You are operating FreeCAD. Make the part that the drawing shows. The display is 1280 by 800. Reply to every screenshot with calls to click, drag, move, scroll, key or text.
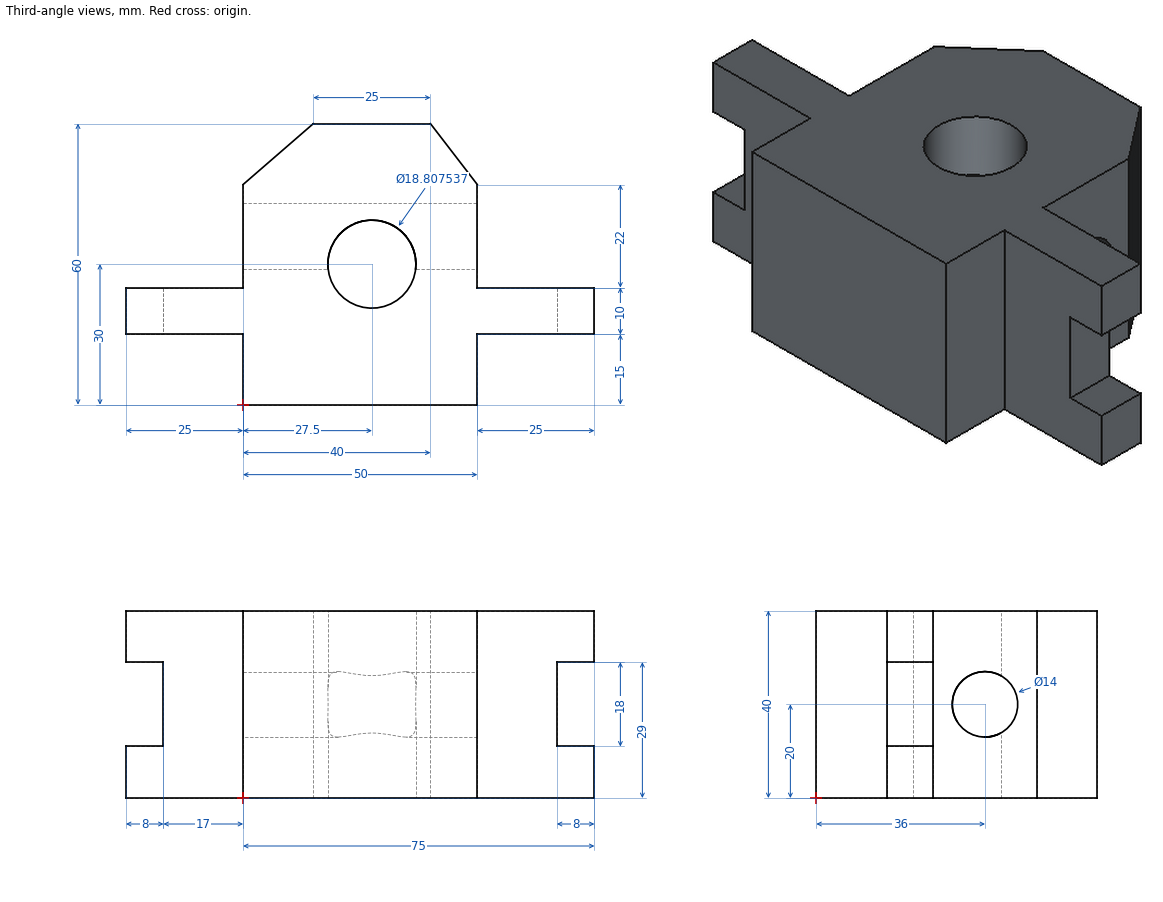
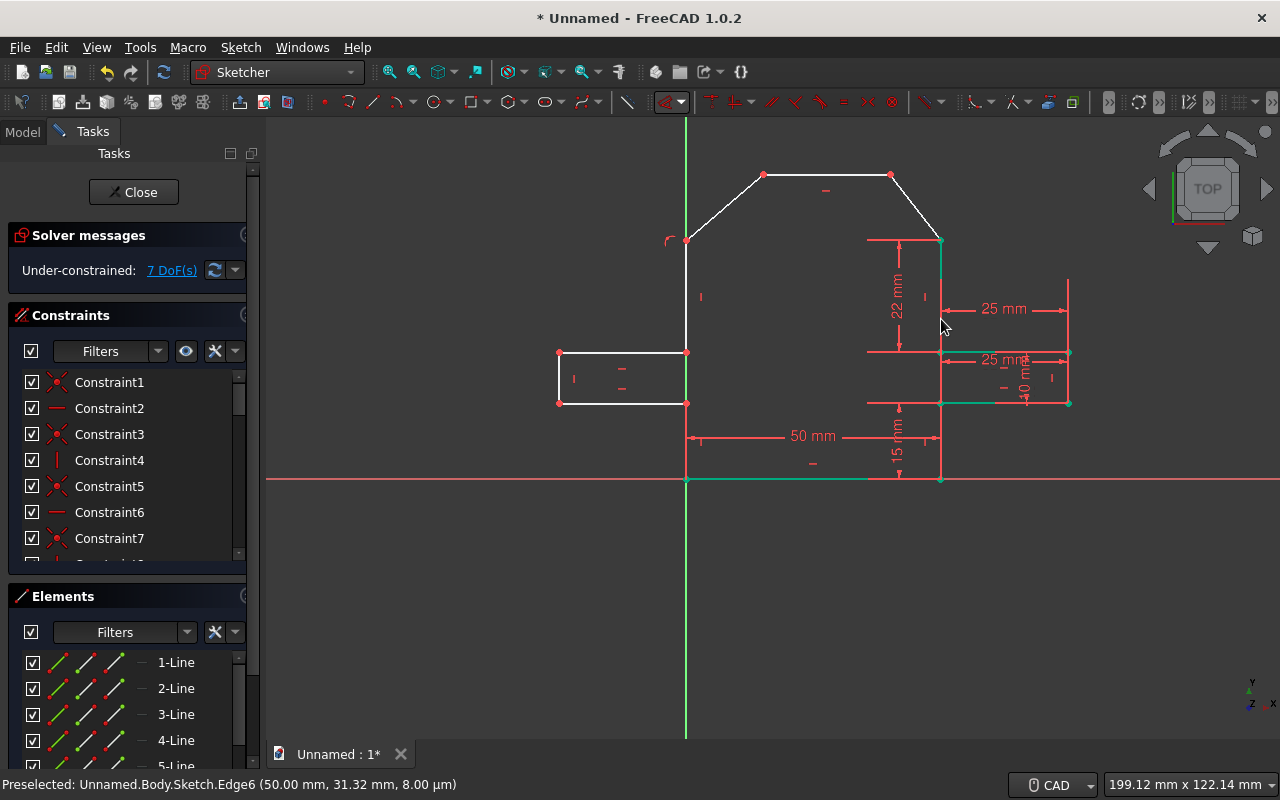
click(852, 175)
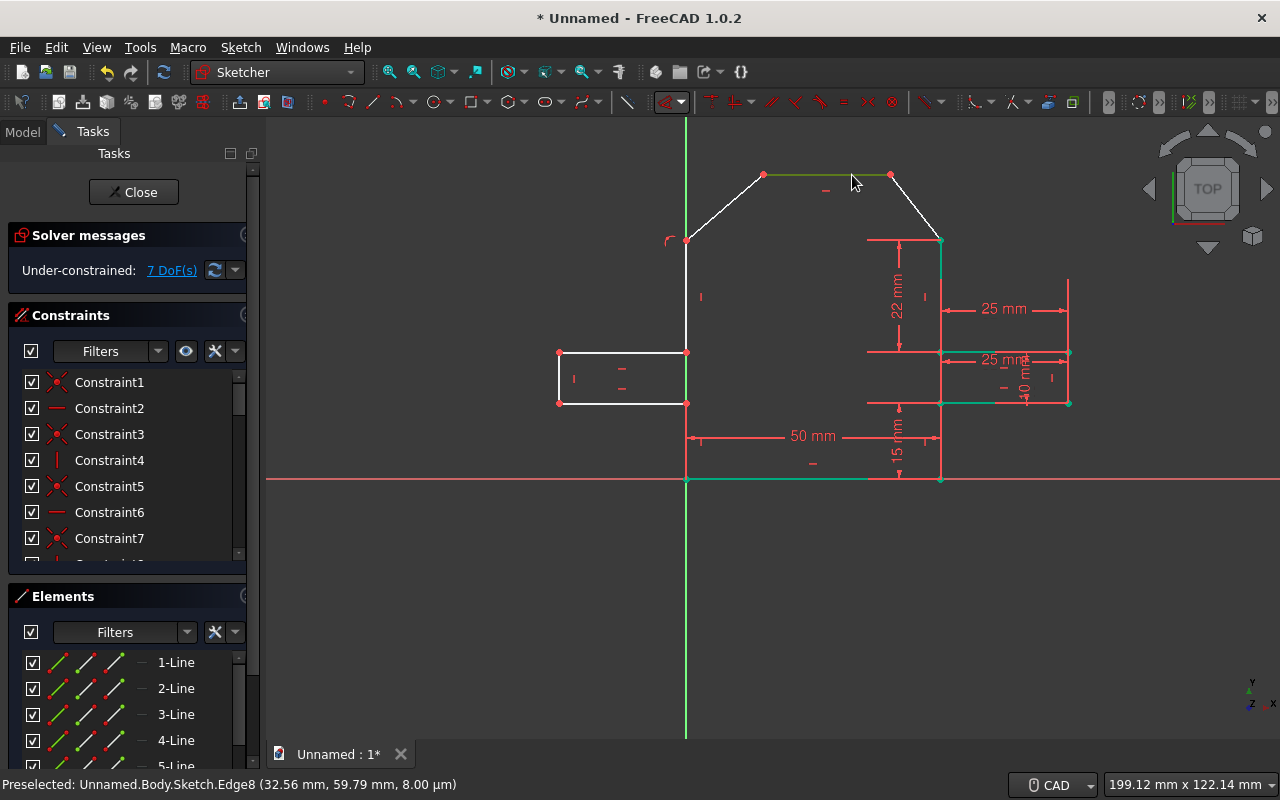
key(l)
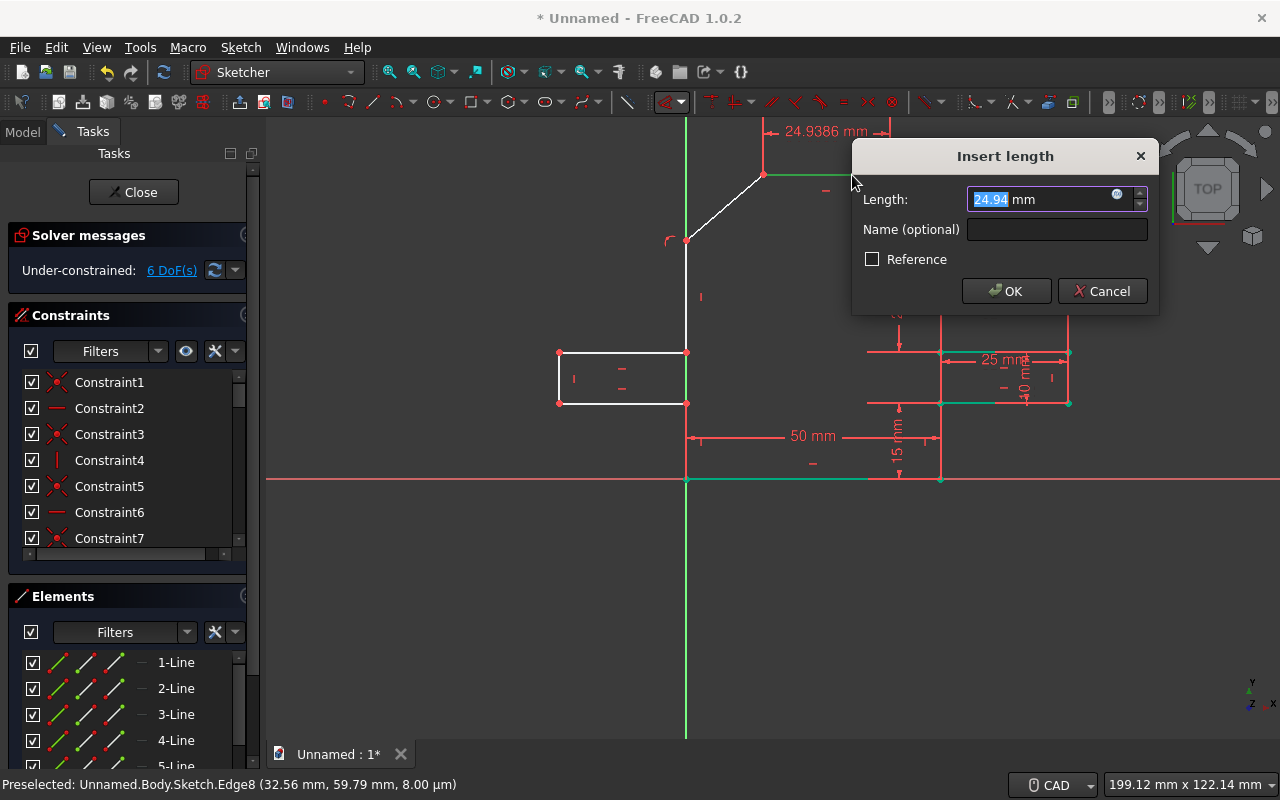
text(25)
key(Return)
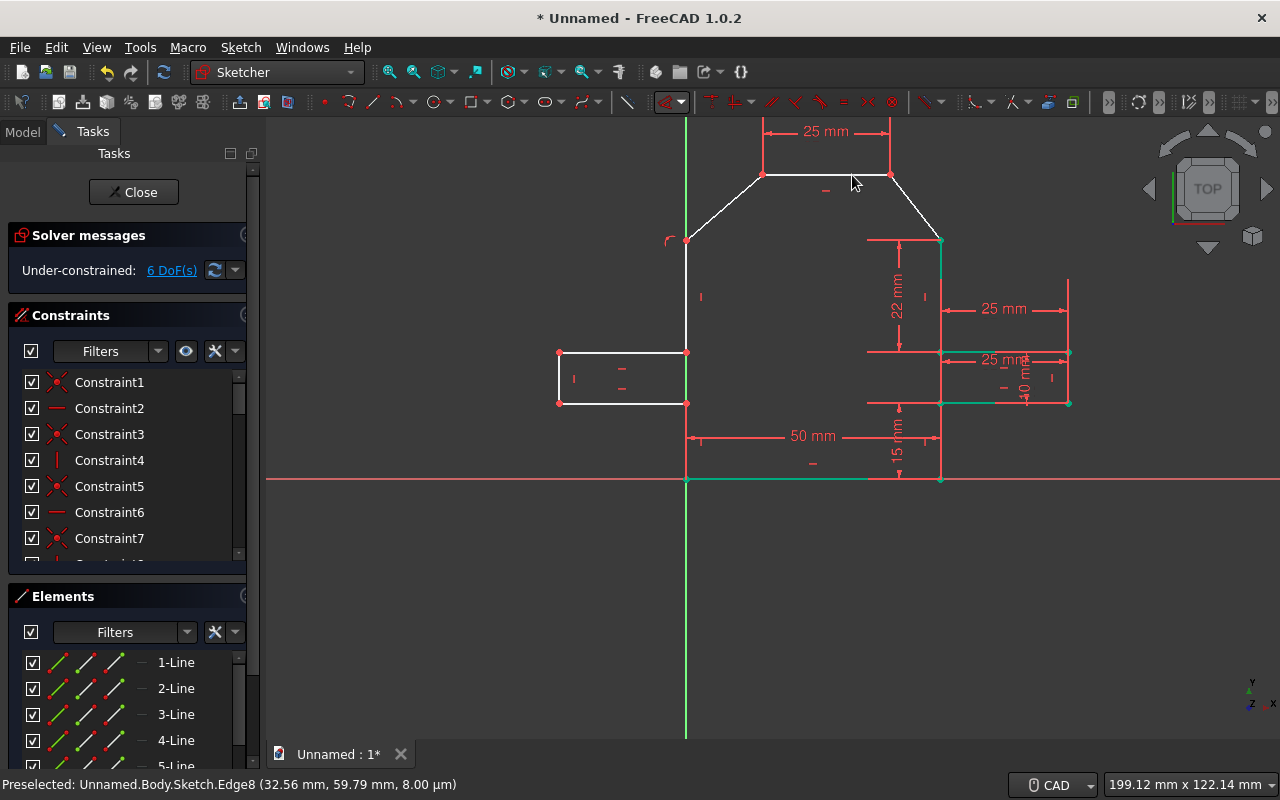
click(686, 275)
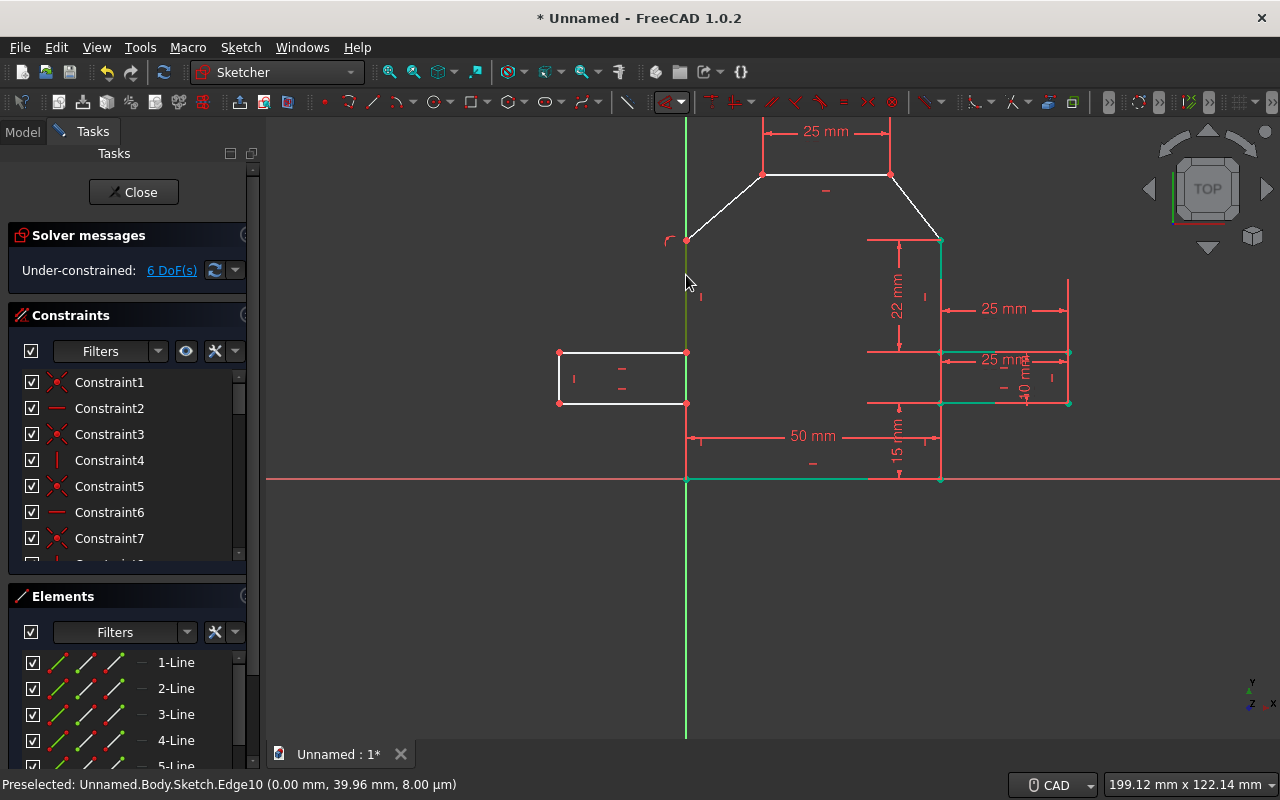
key(i)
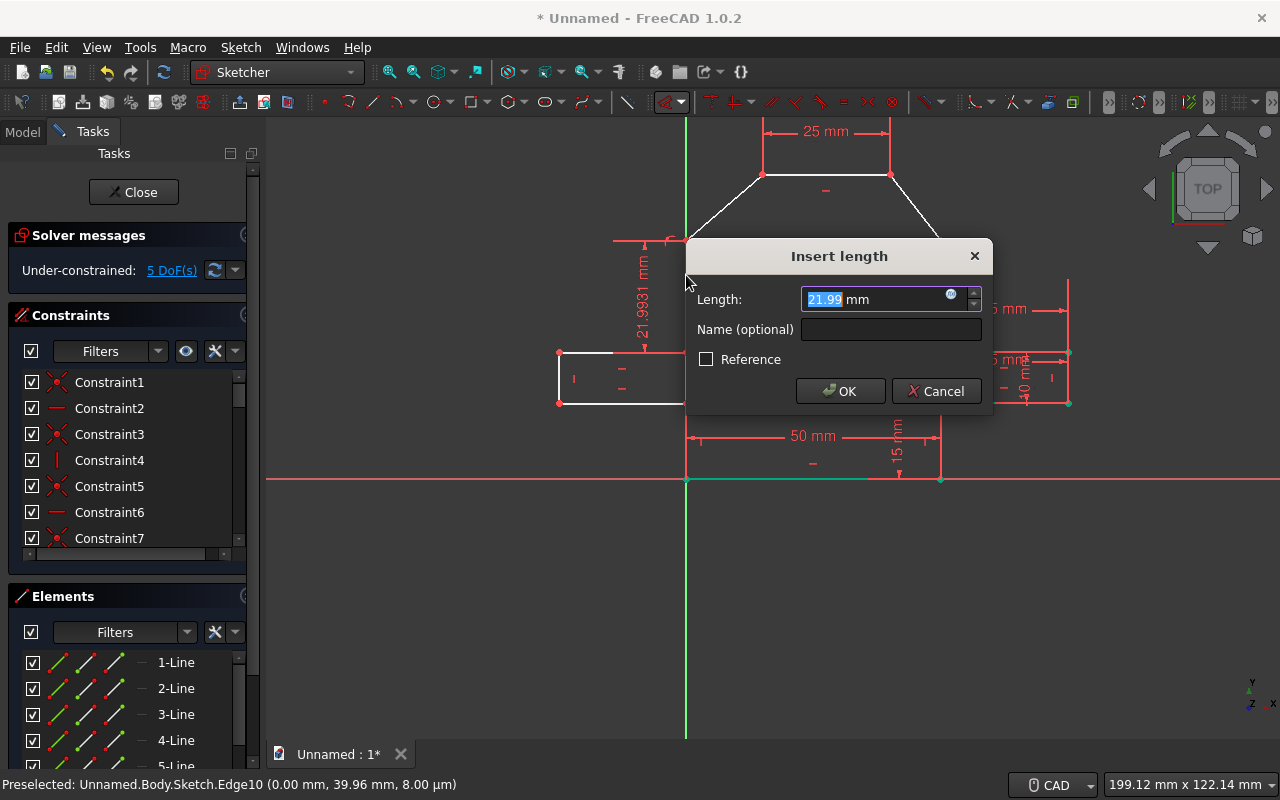
text(22)
key(Return)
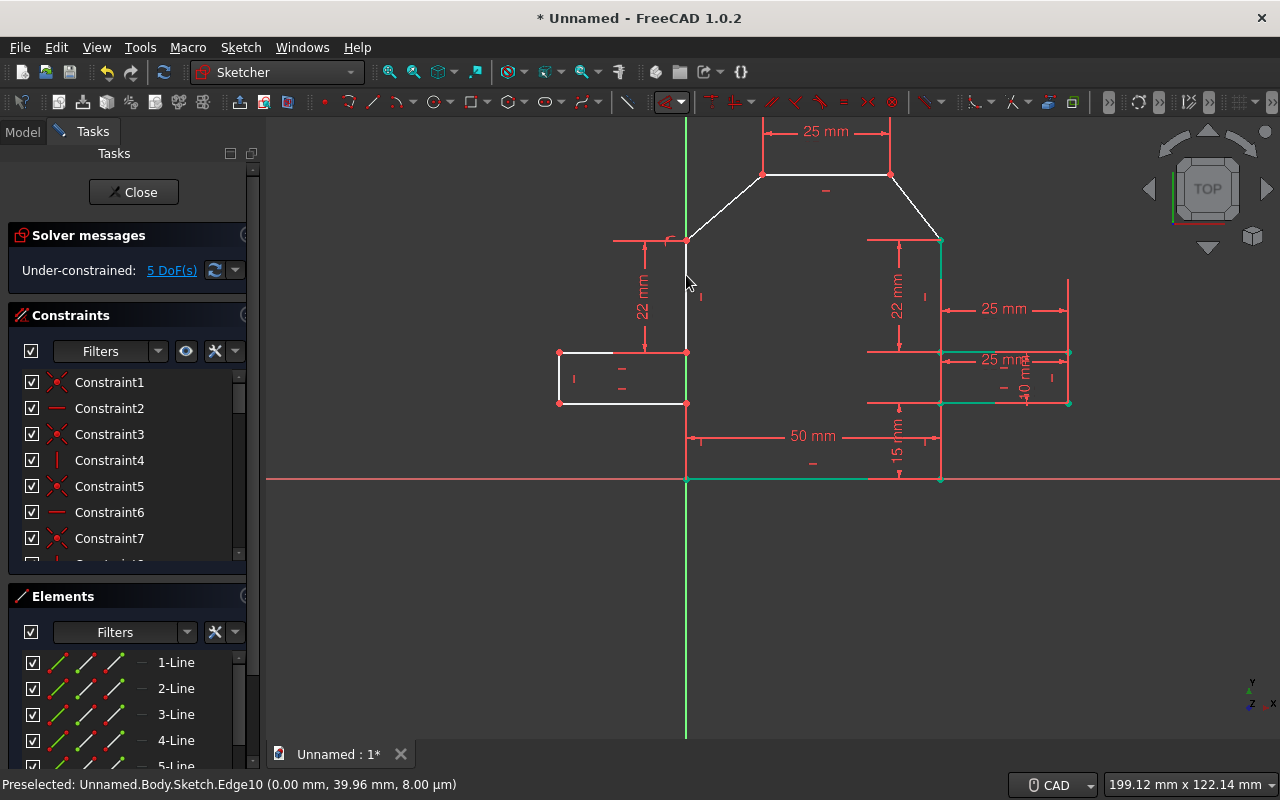
click(648, 353)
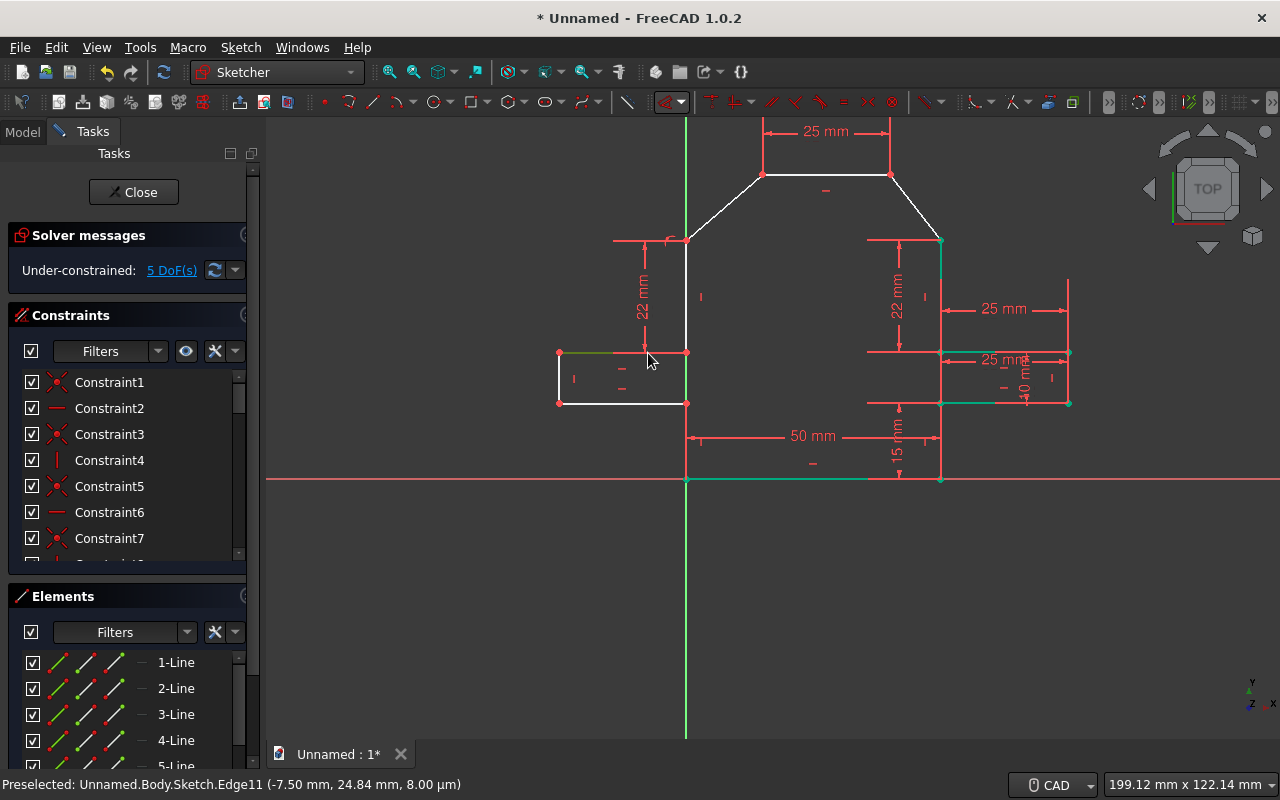
key(l)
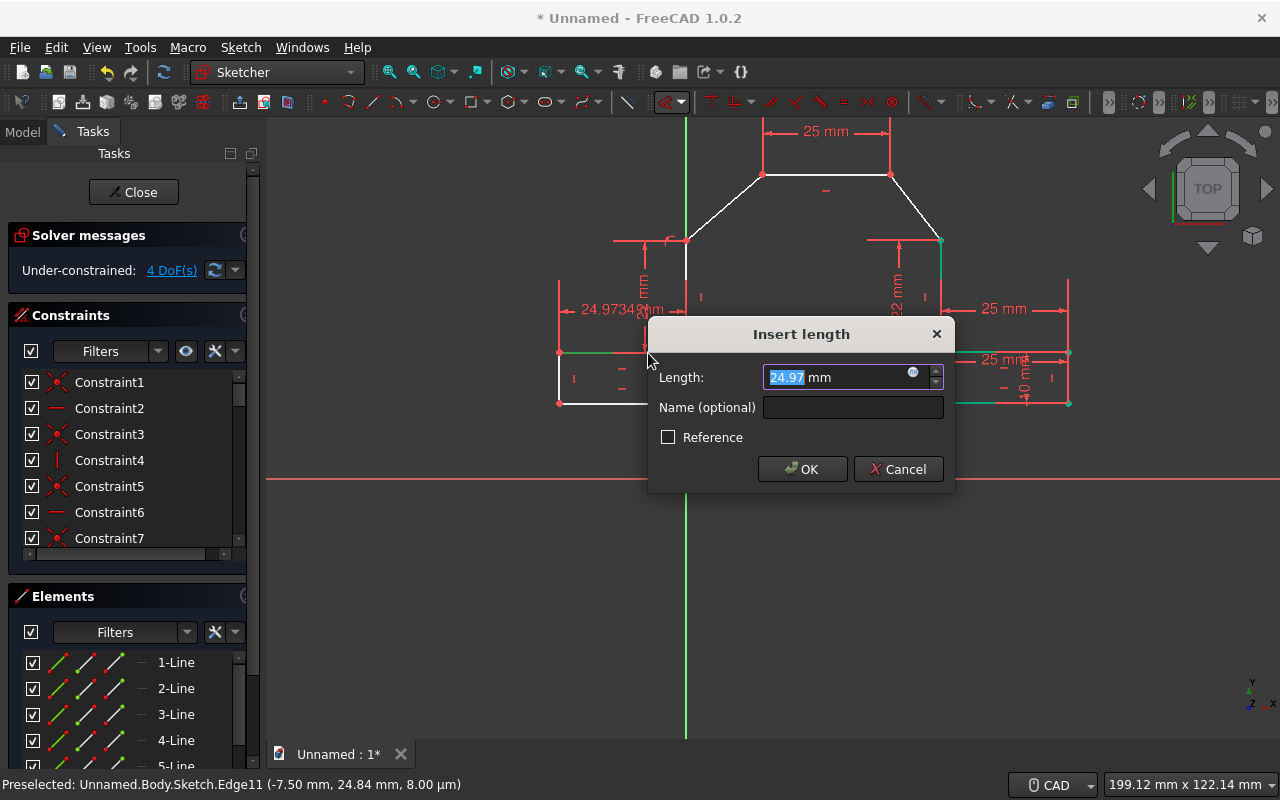
text(25)
key(Return)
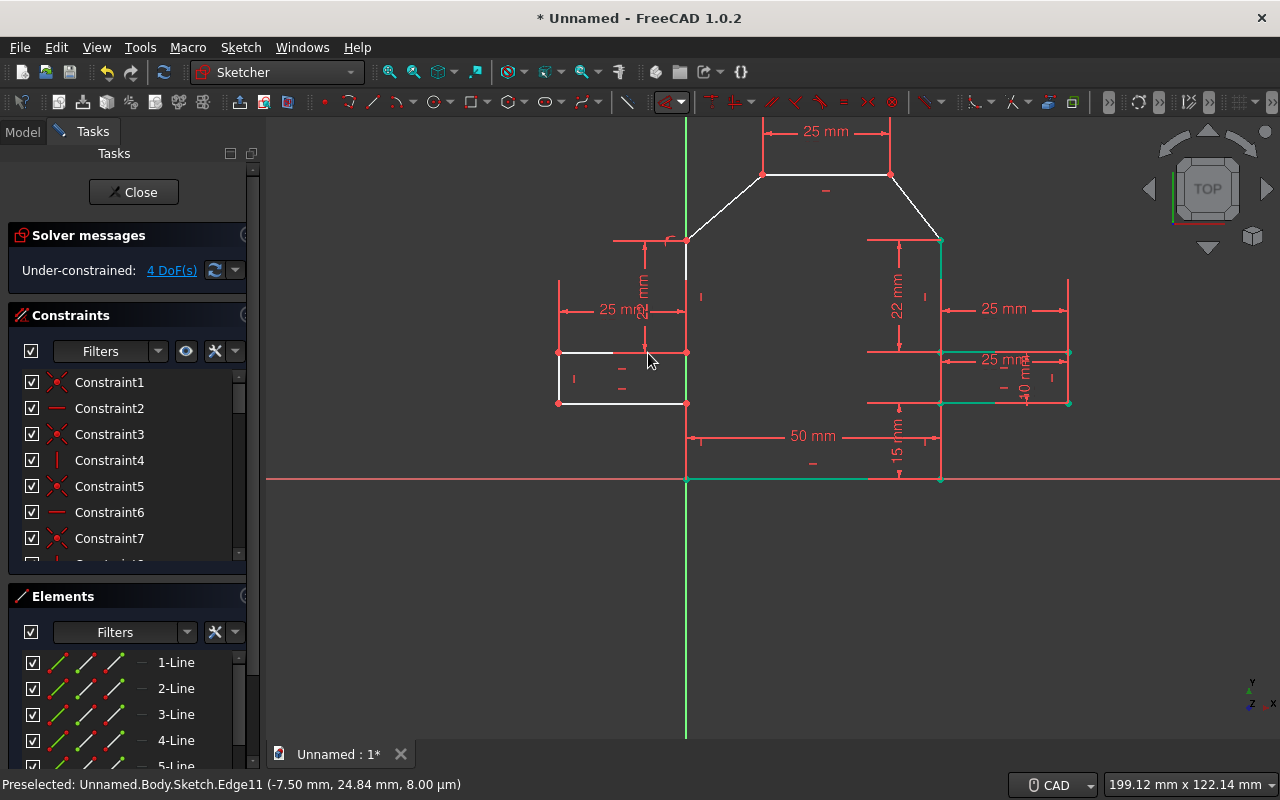
click(559, 368)